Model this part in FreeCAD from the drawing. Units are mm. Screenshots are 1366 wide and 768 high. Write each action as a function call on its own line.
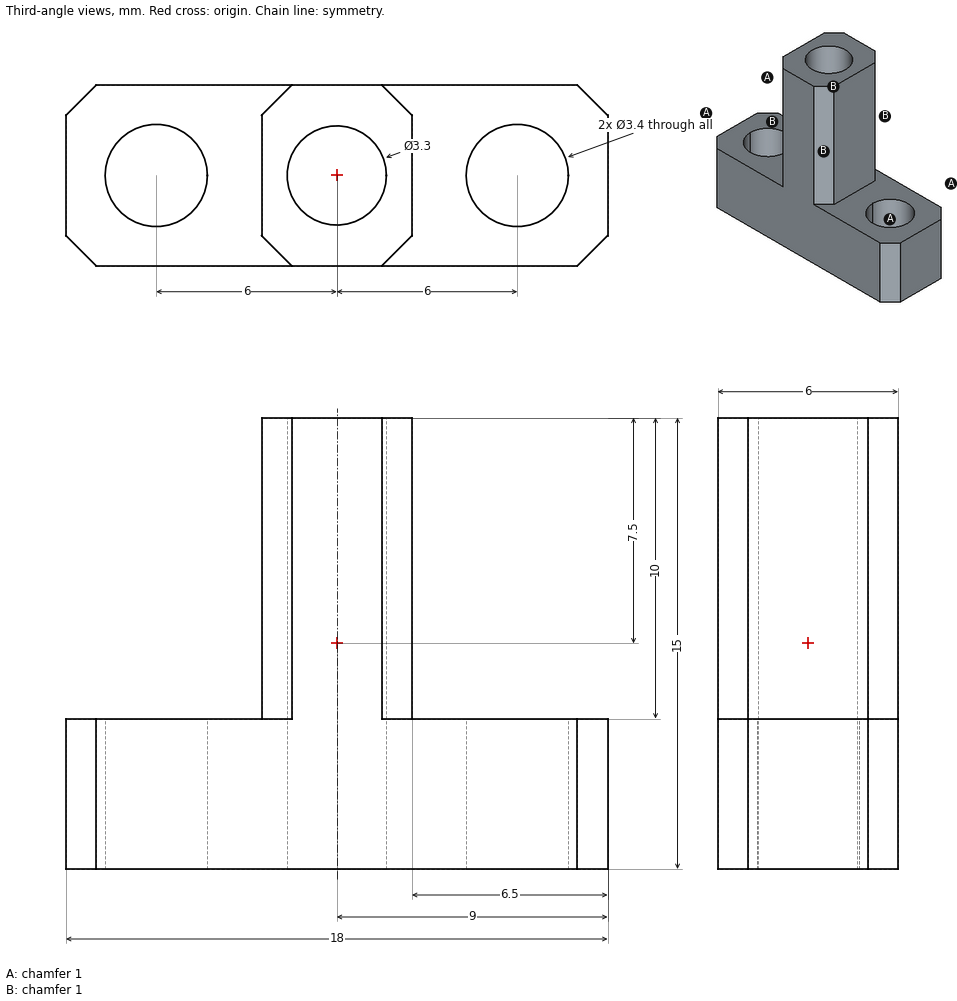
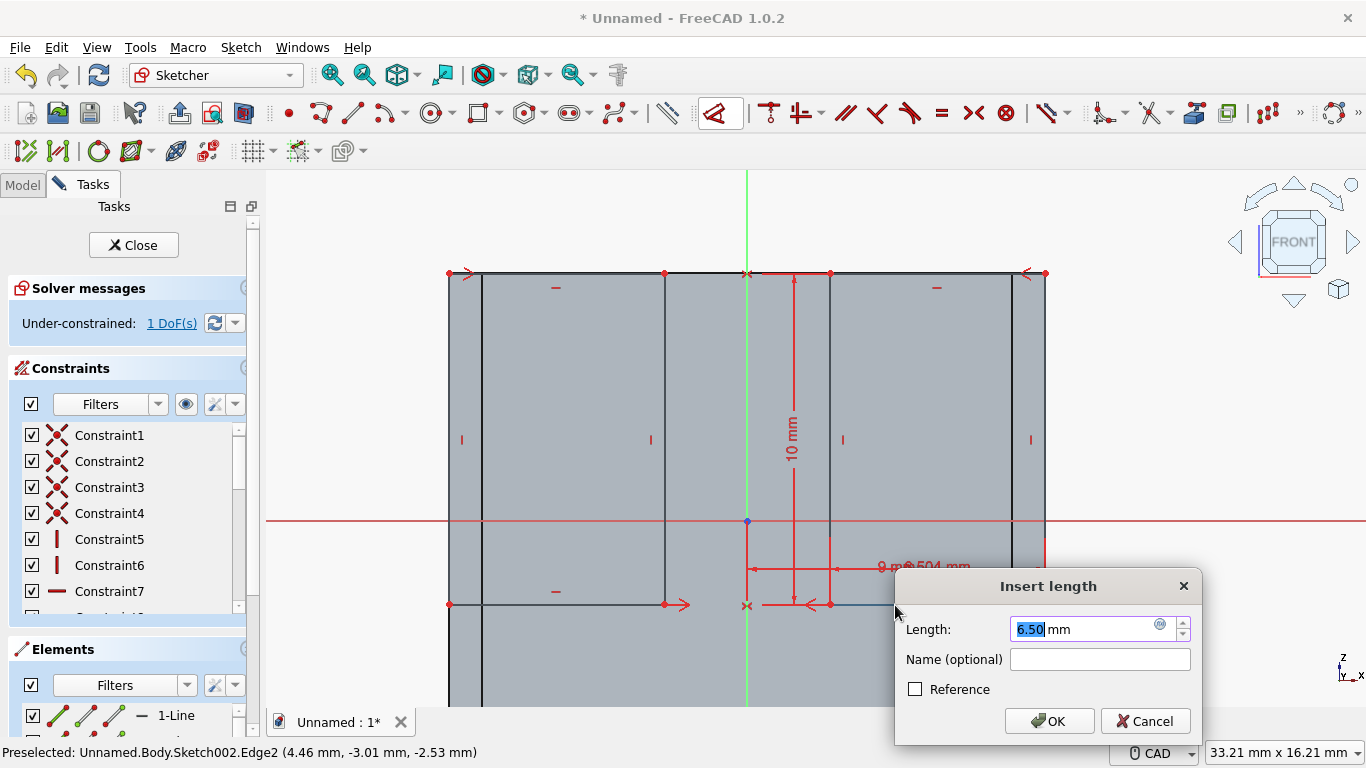
text(6.5)
key(Return)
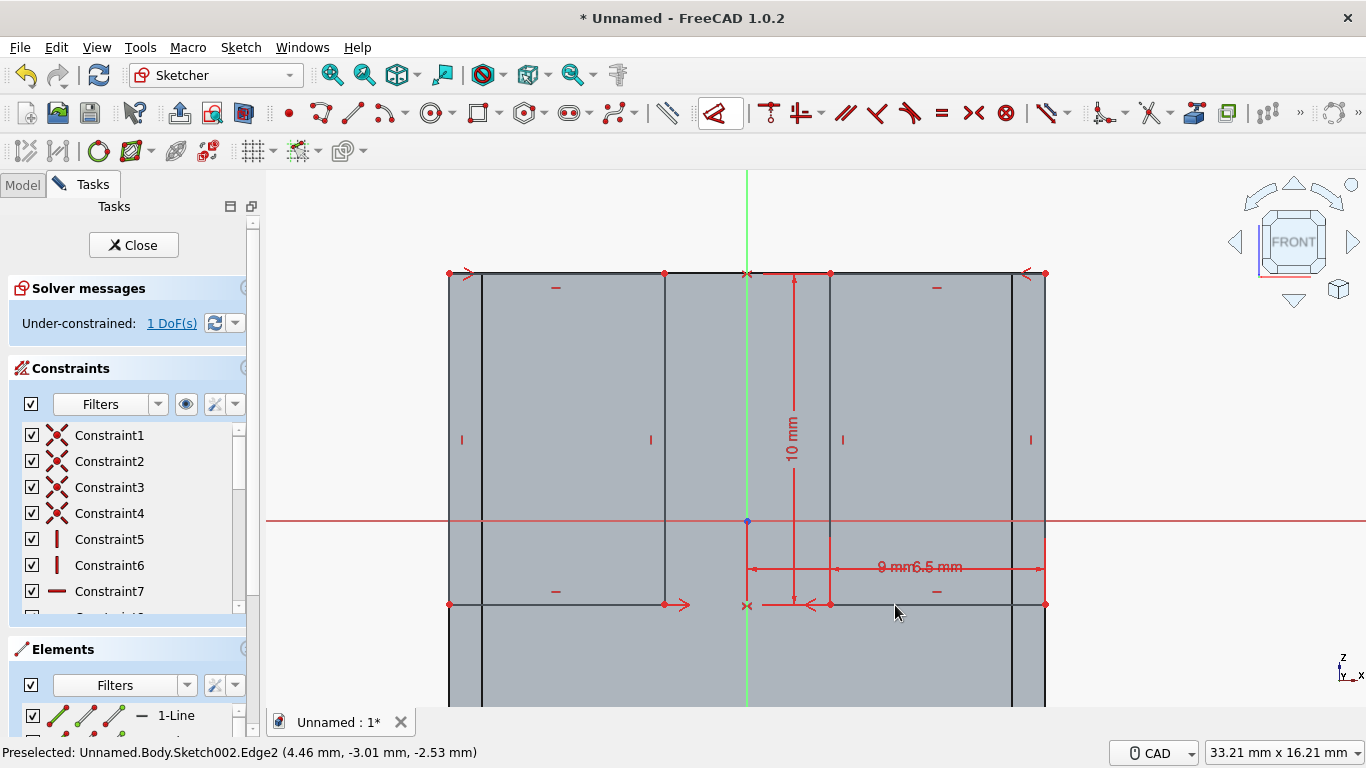
click(830, 274)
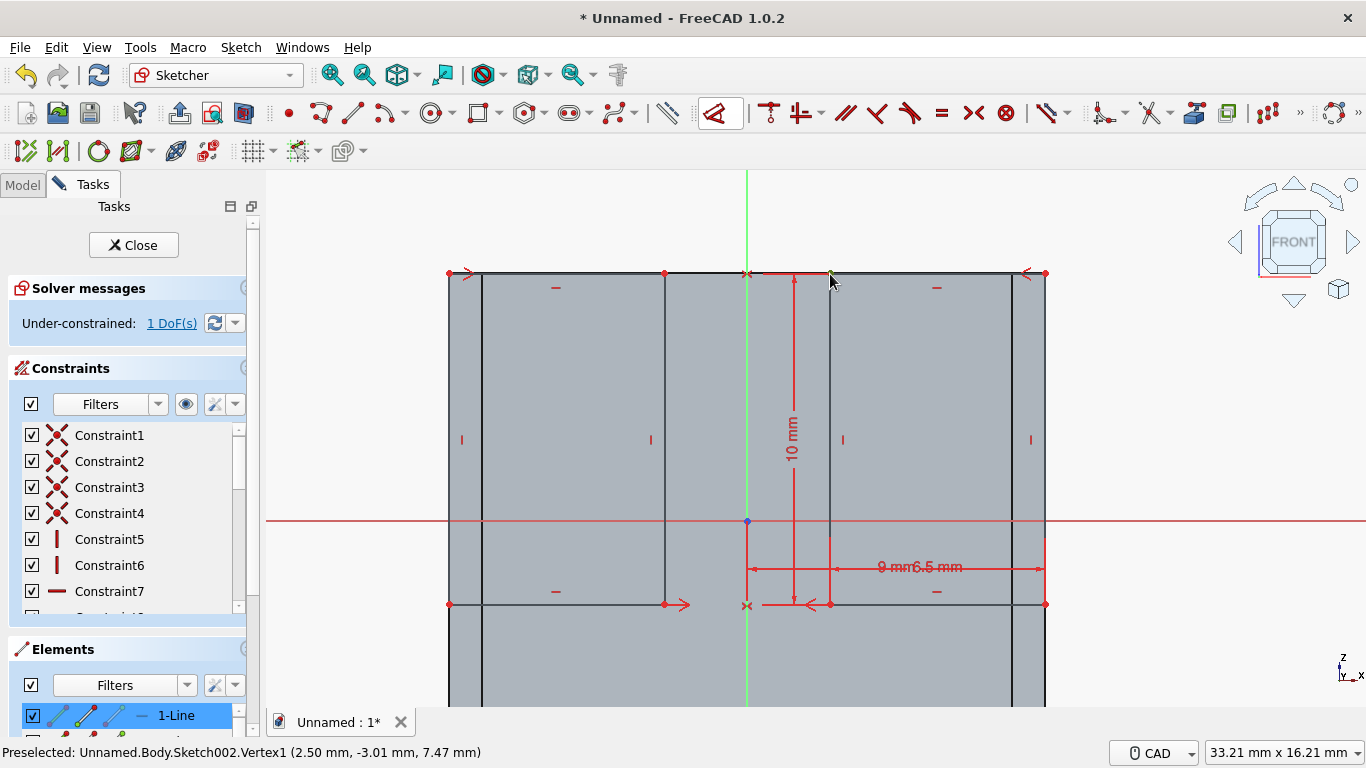
click(738, 114)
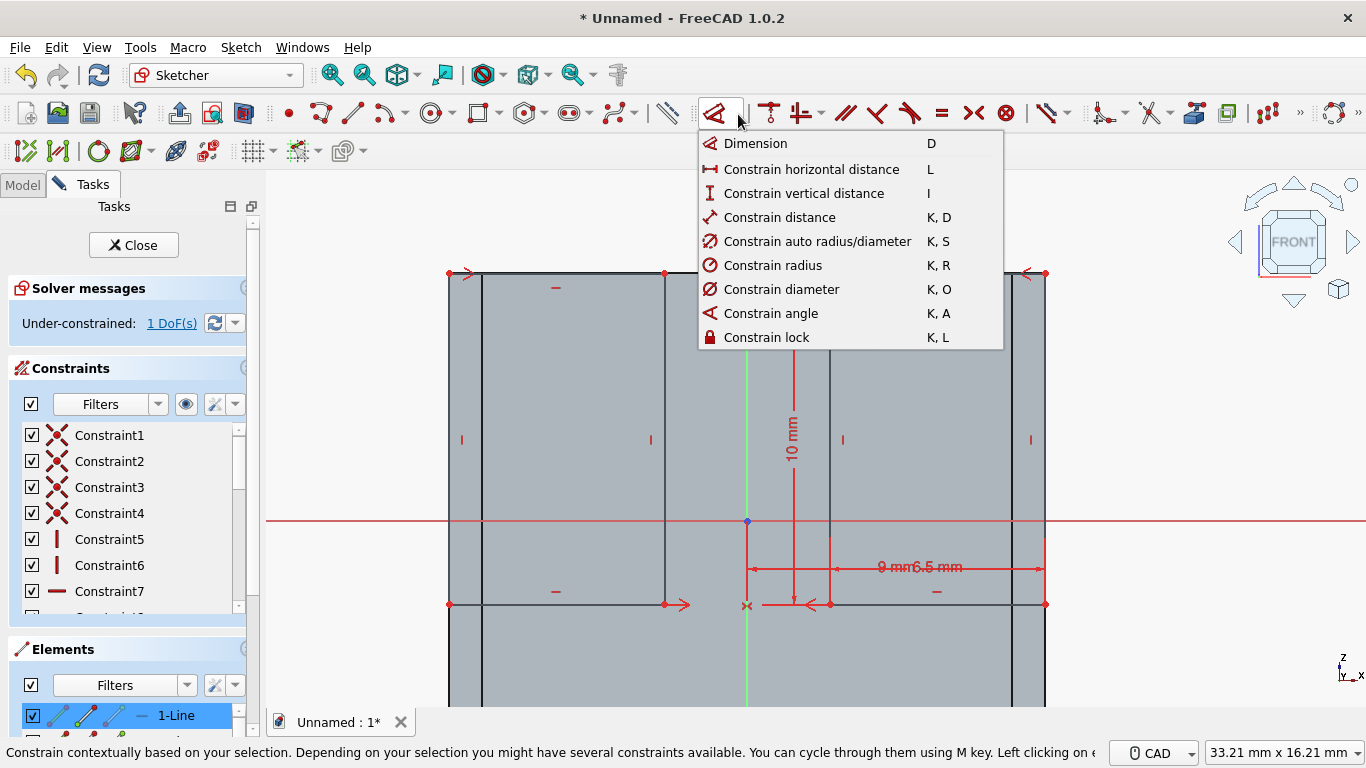
click(851, 193)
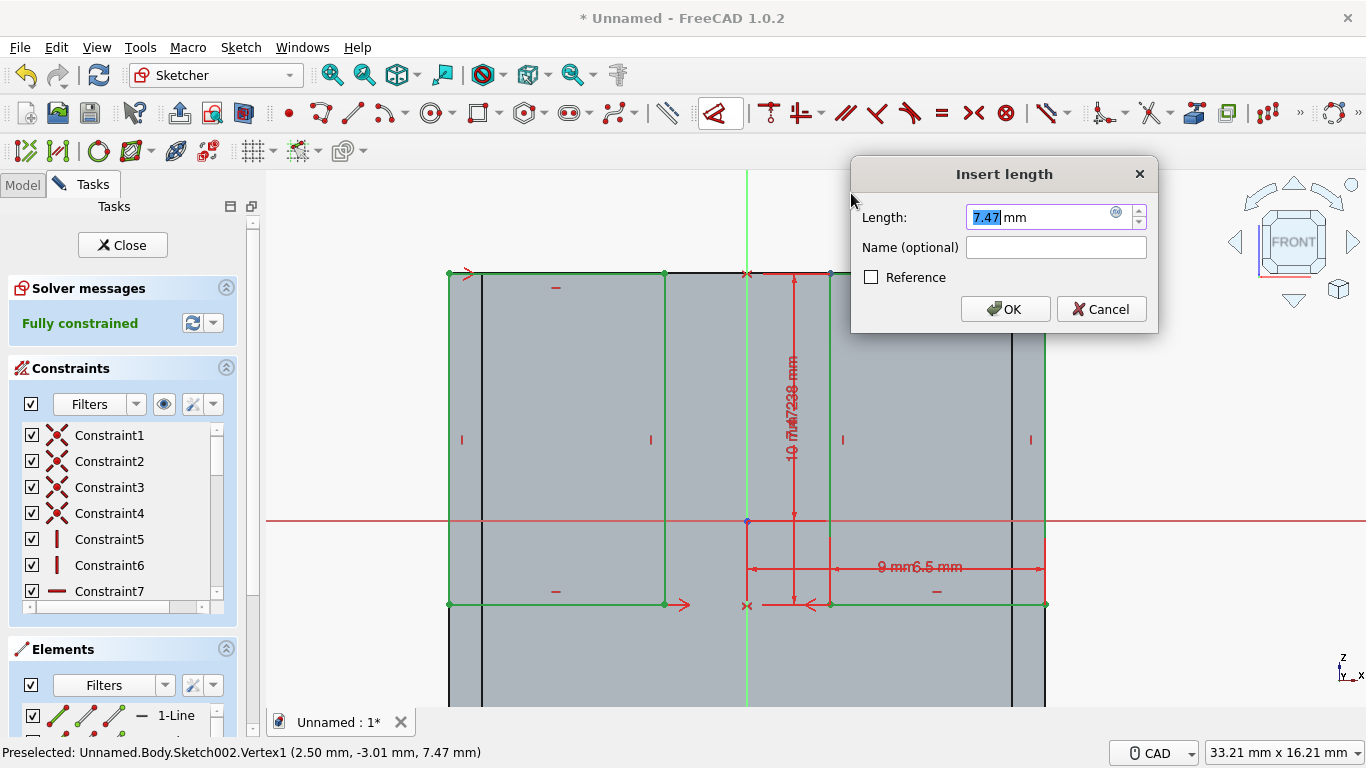
text(7.5)
key(Return)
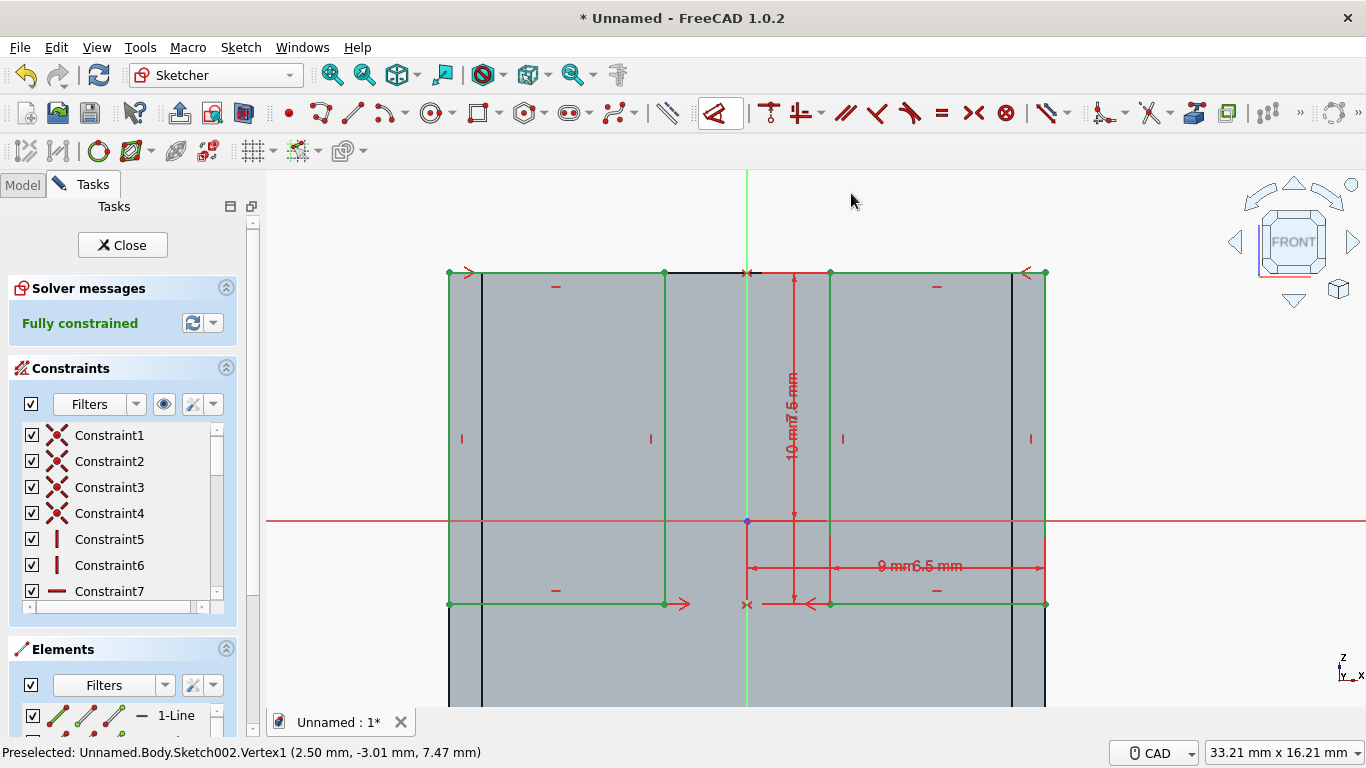
click(123, 245)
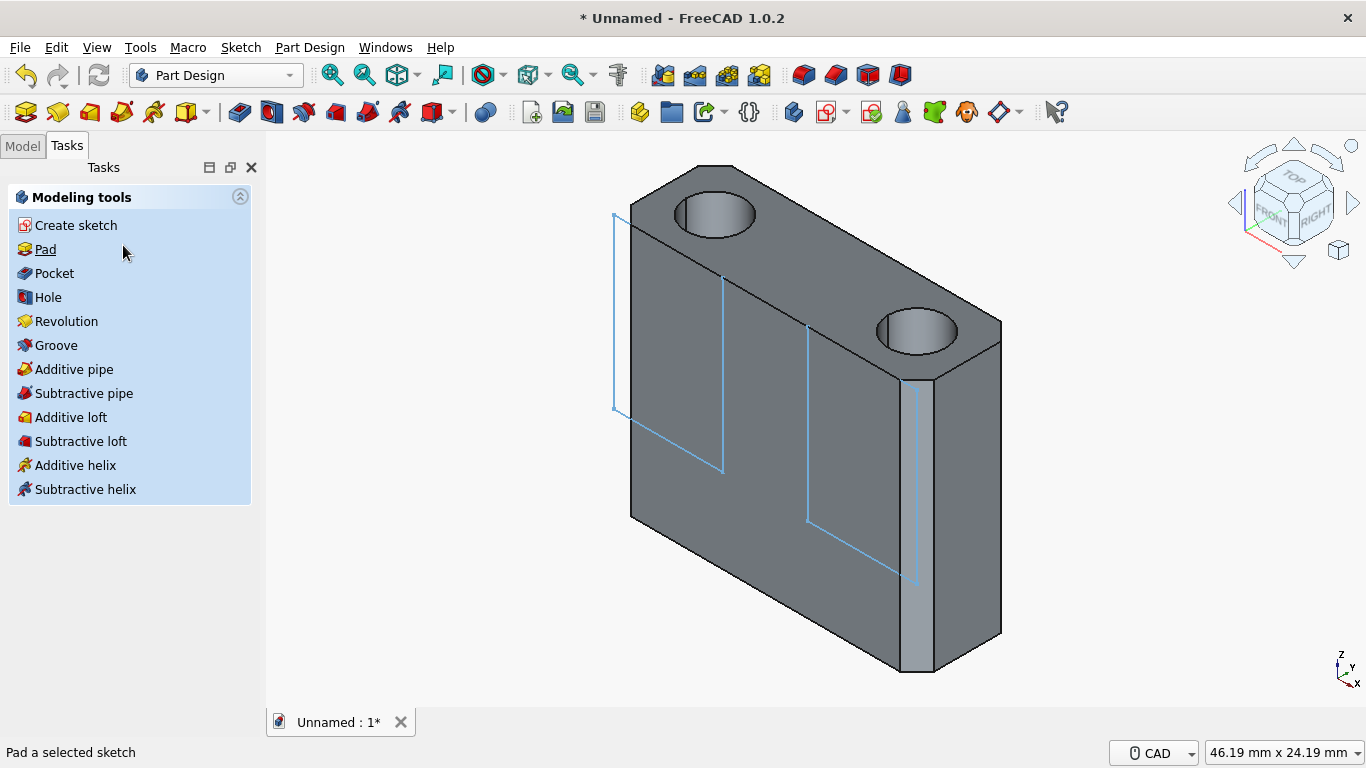
click(240, 112)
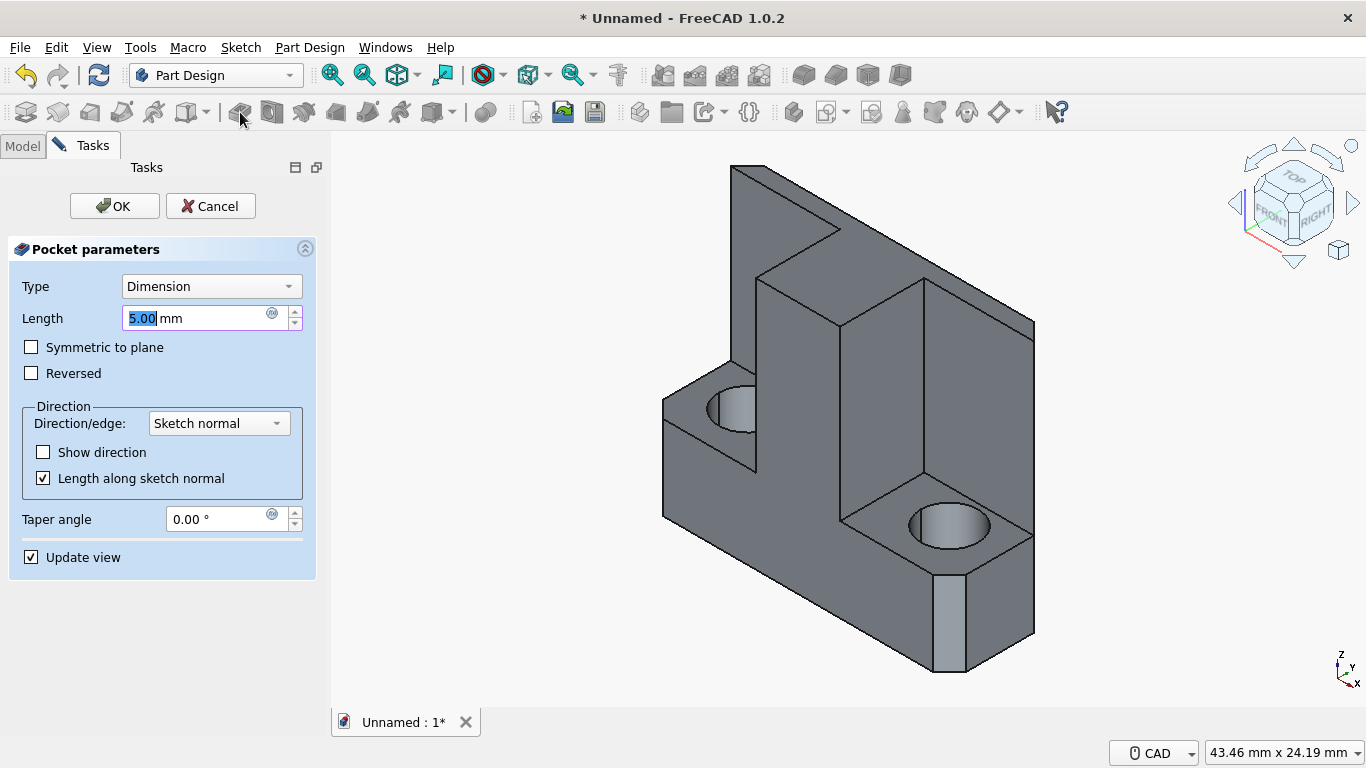
click(212, 286)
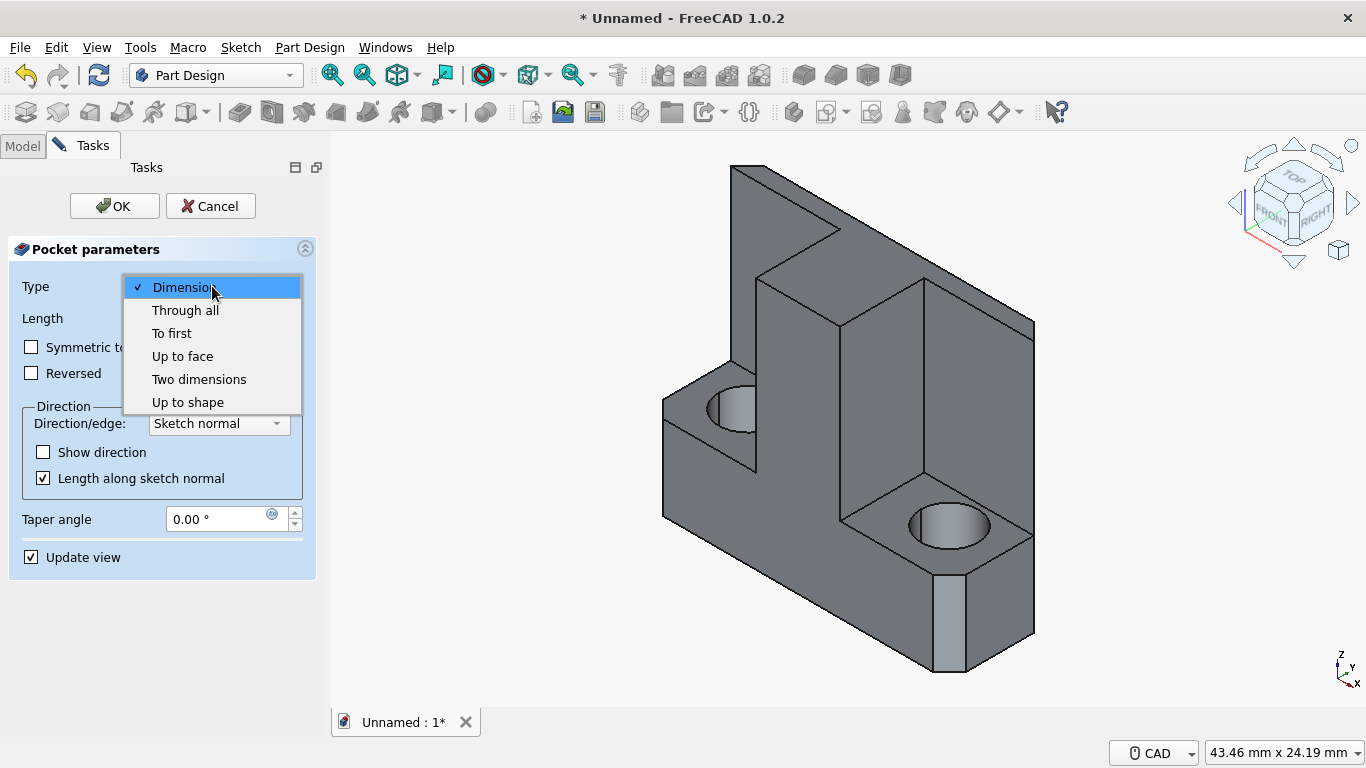
click(212, 310)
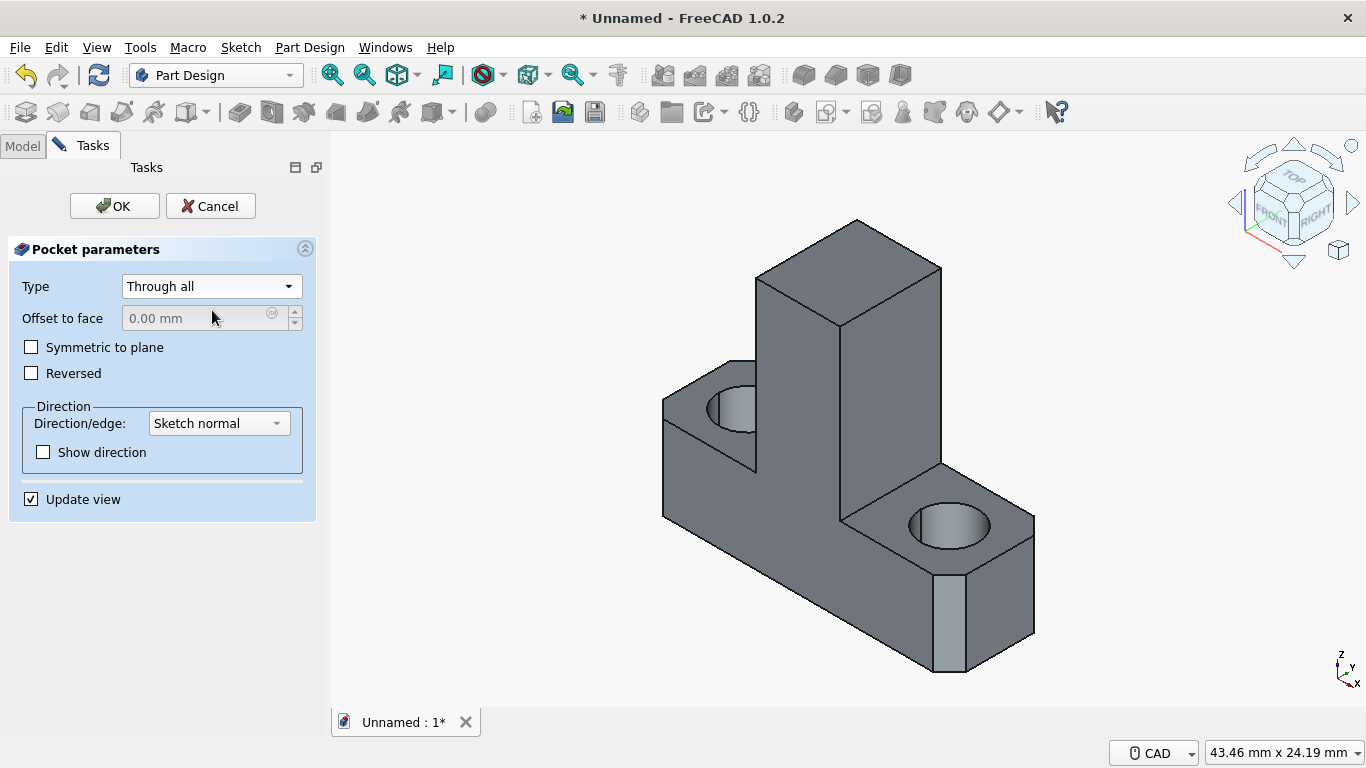
click(115, 206)